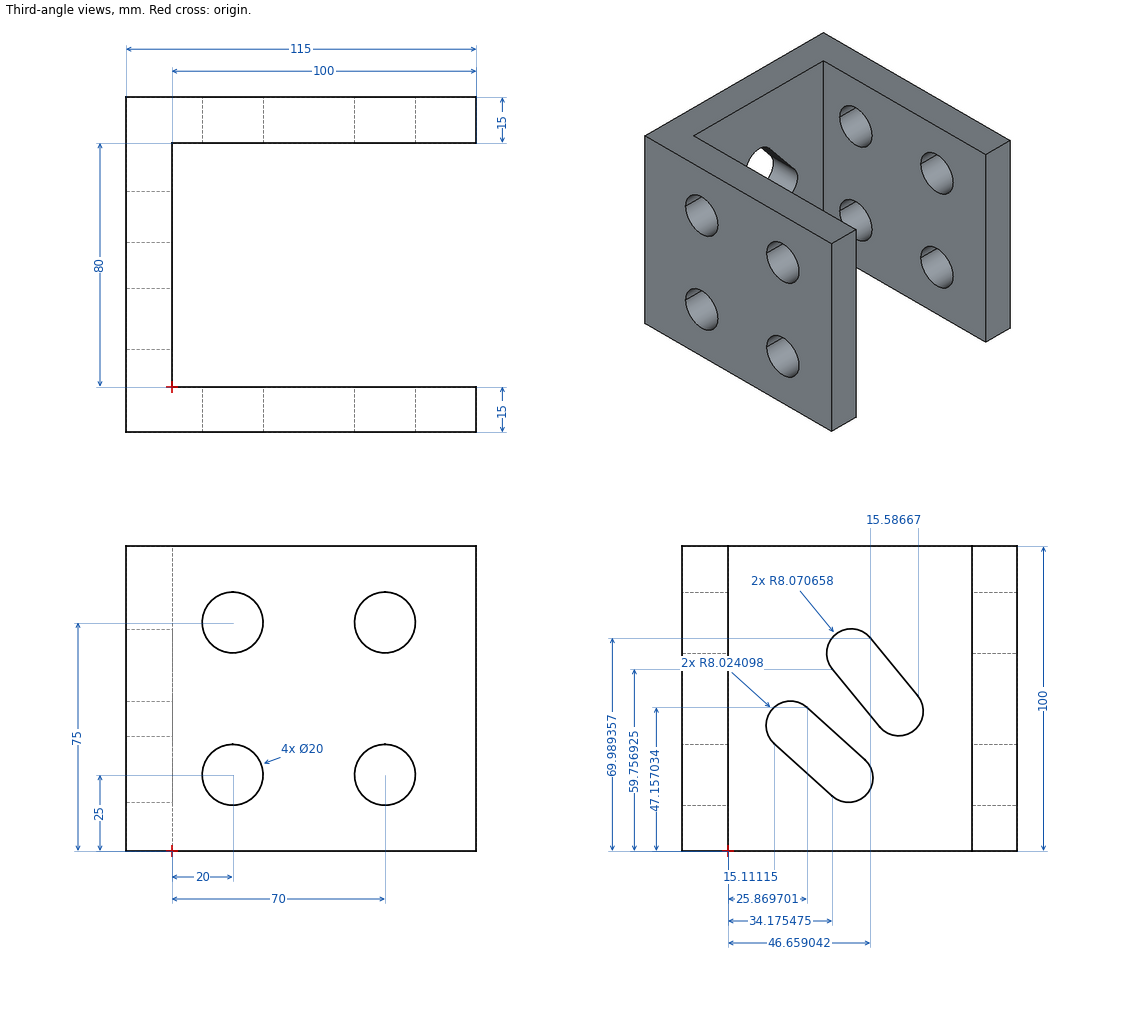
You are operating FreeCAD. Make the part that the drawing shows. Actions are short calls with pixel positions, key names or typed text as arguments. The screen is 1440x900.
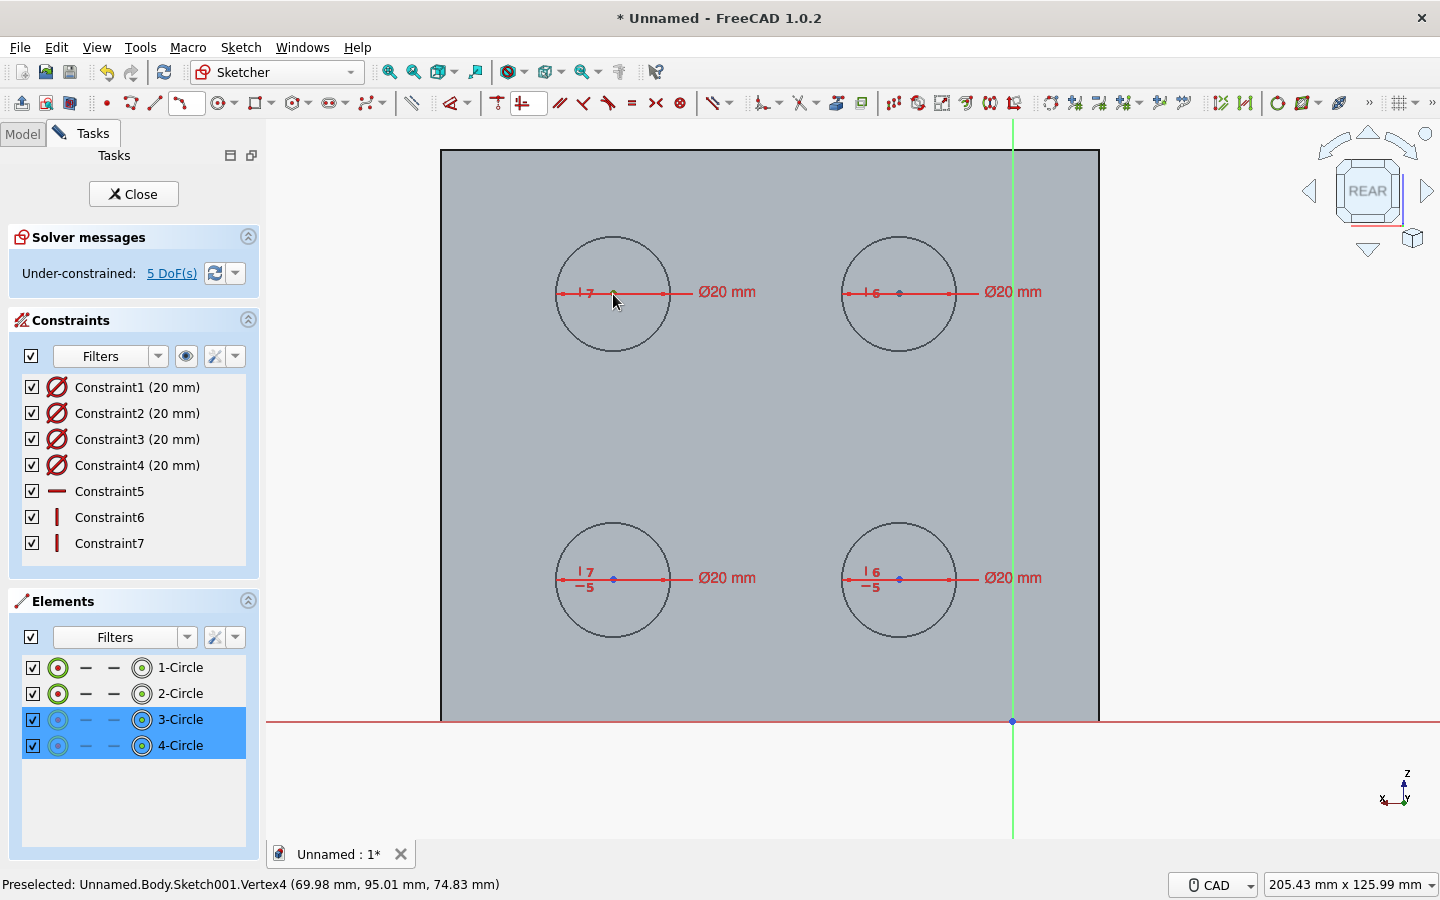
key(h)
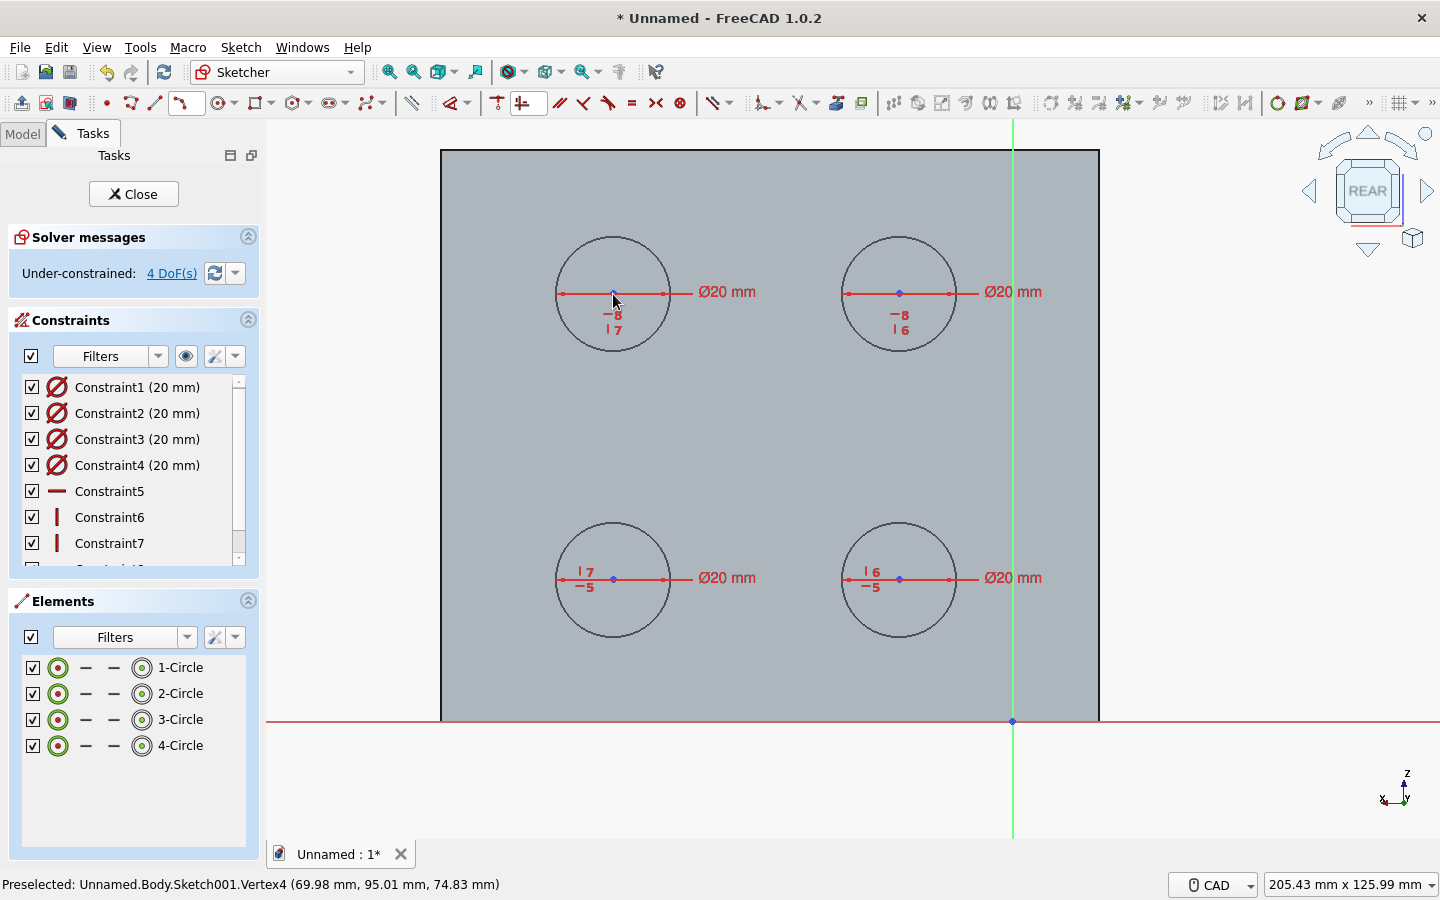
key(d)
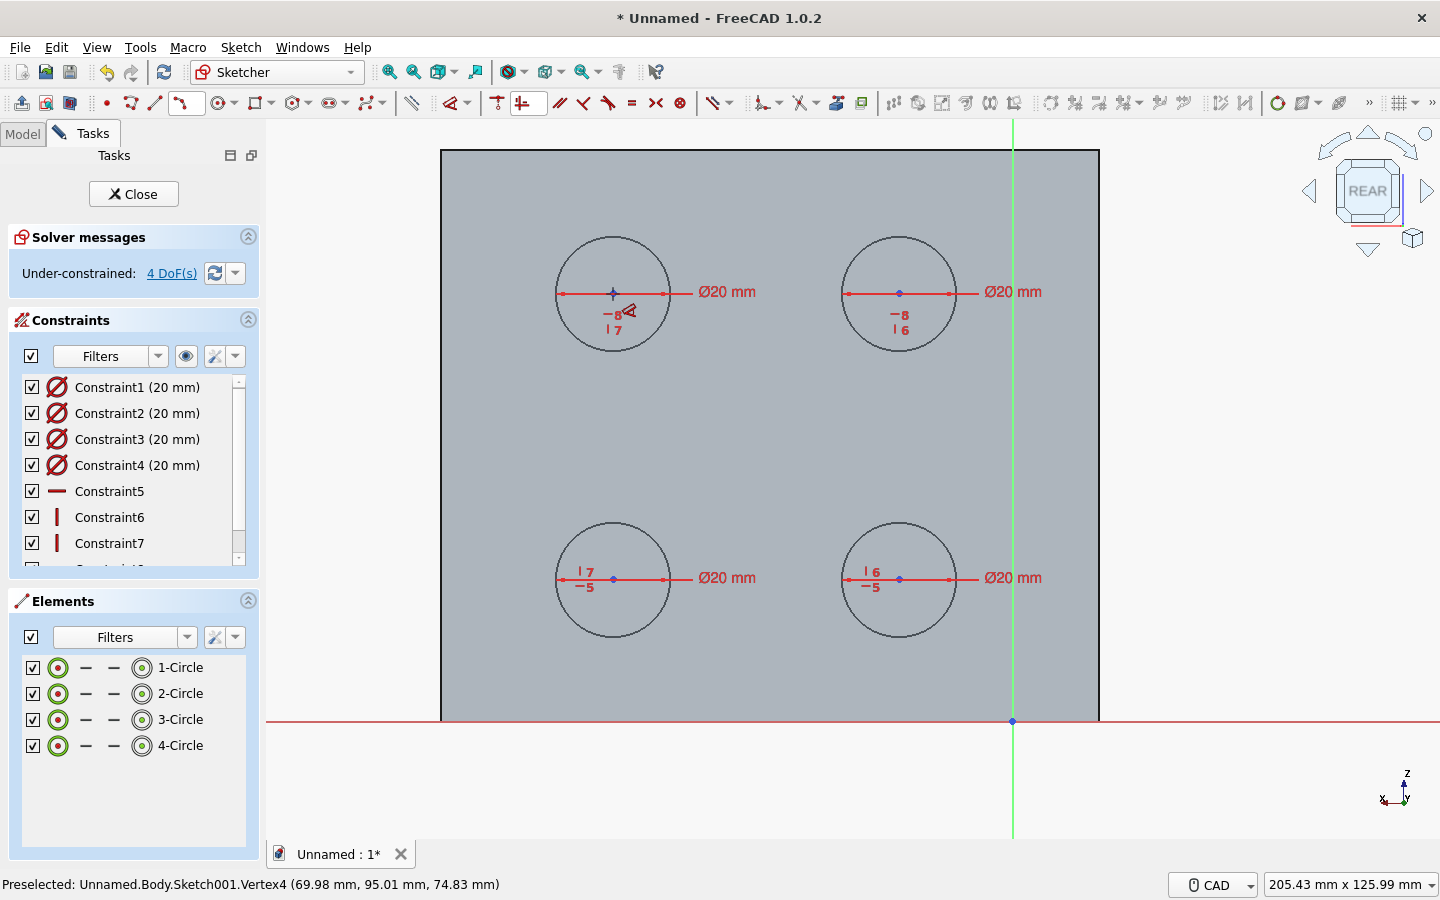
click(899, 580)
click(956, 756)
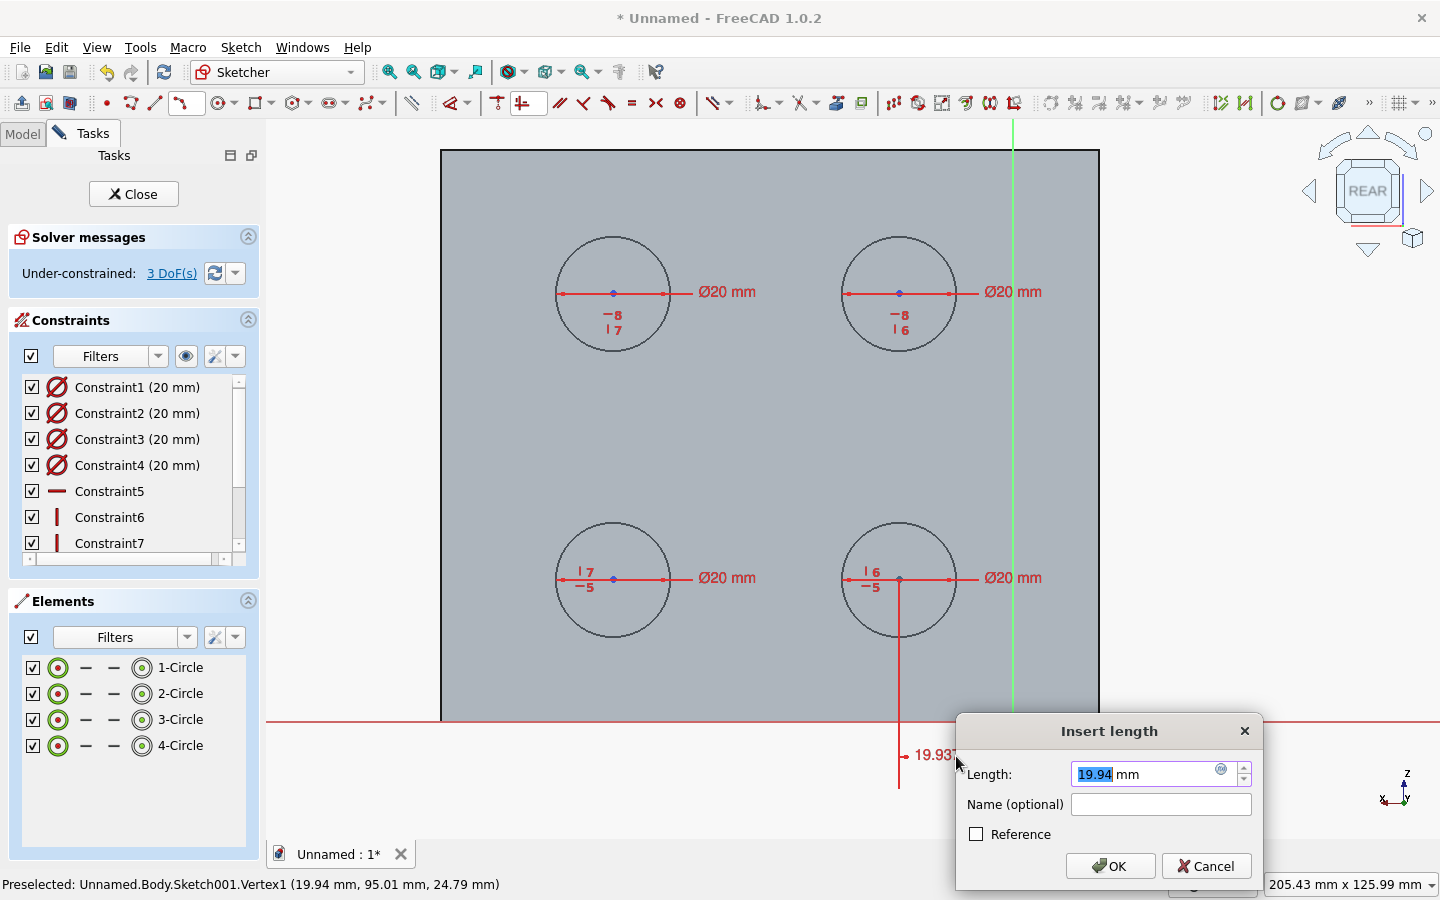
text(20)
key(Return)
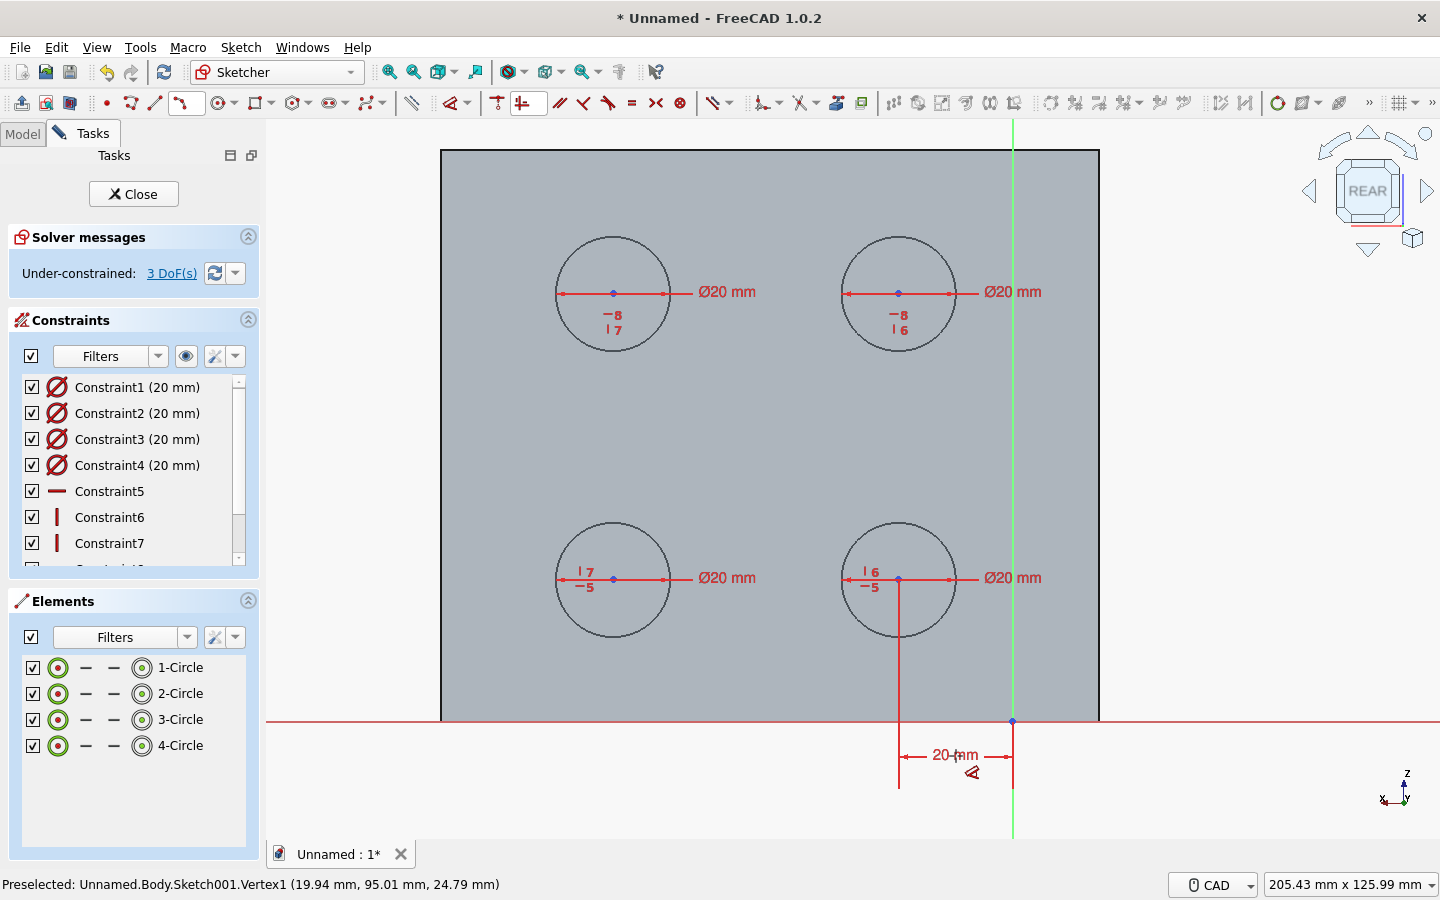
click(899, 580)
click(1047, 651)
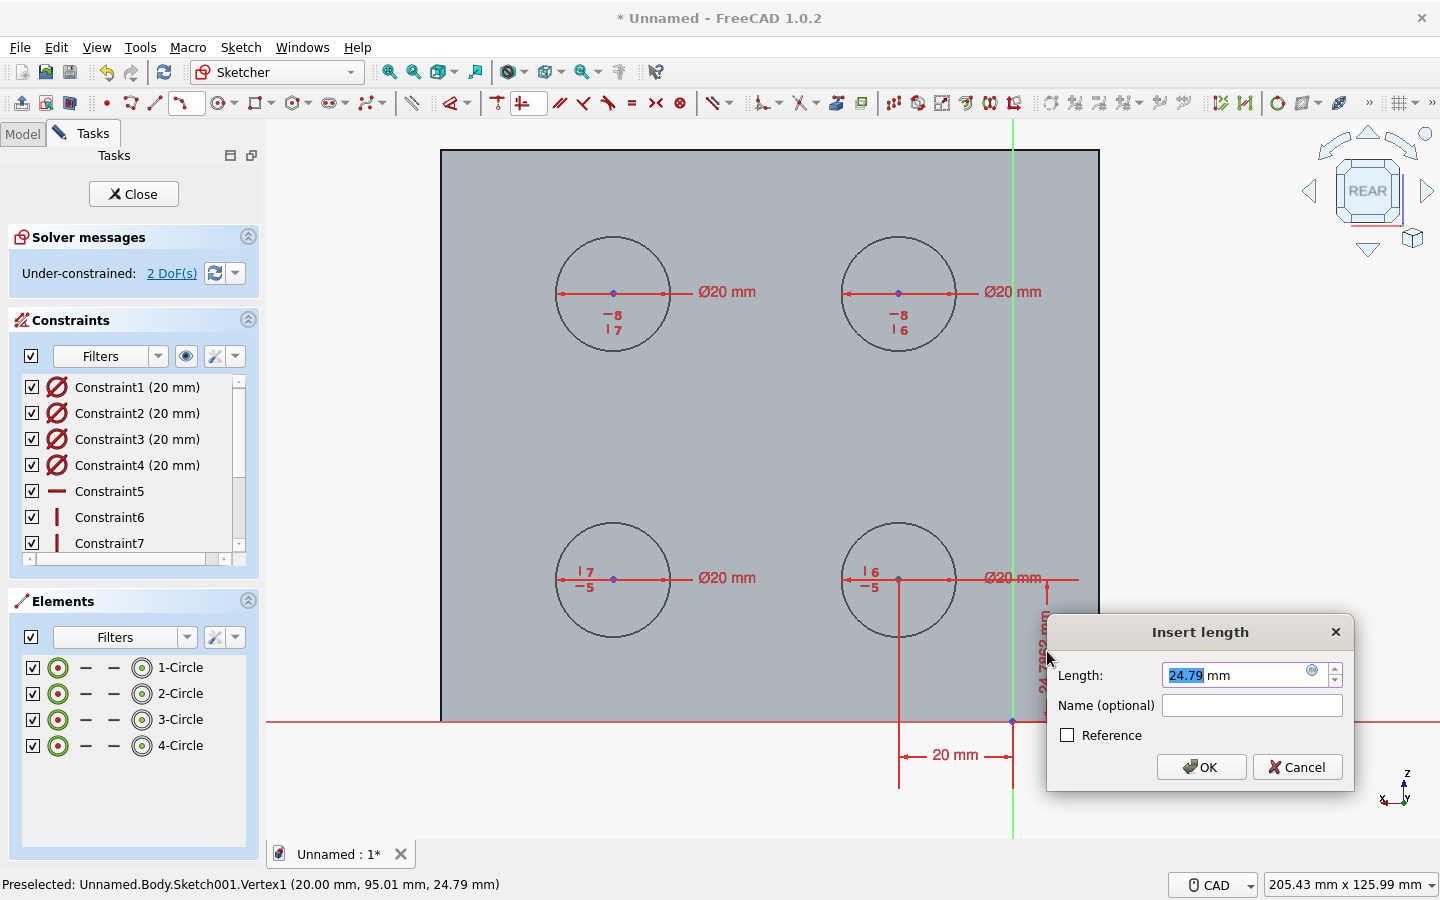
text(25)
key(Return)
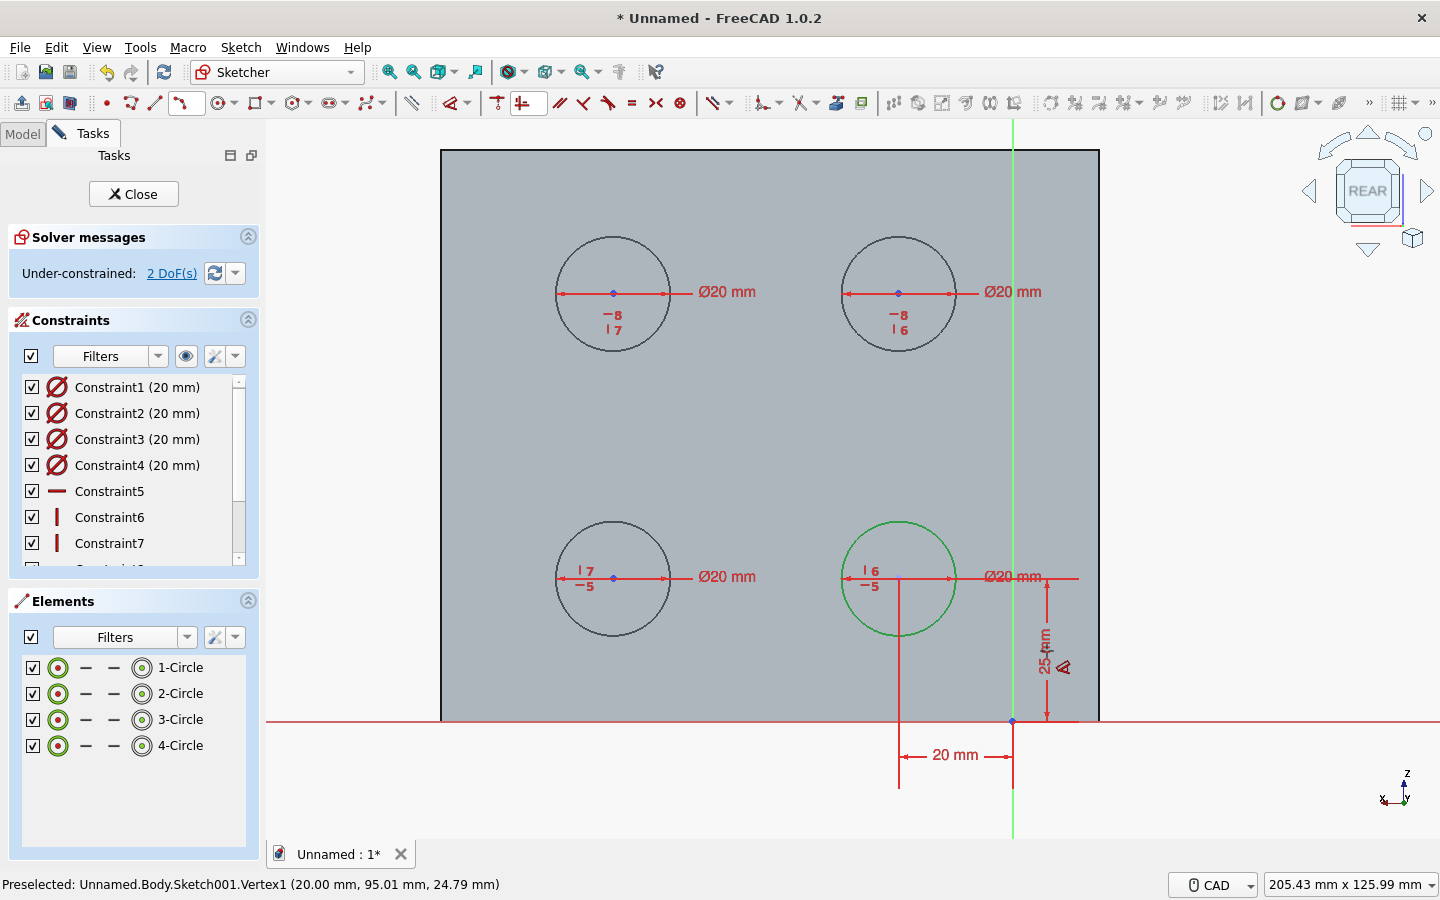
click(613, 579)
click(813, 756)